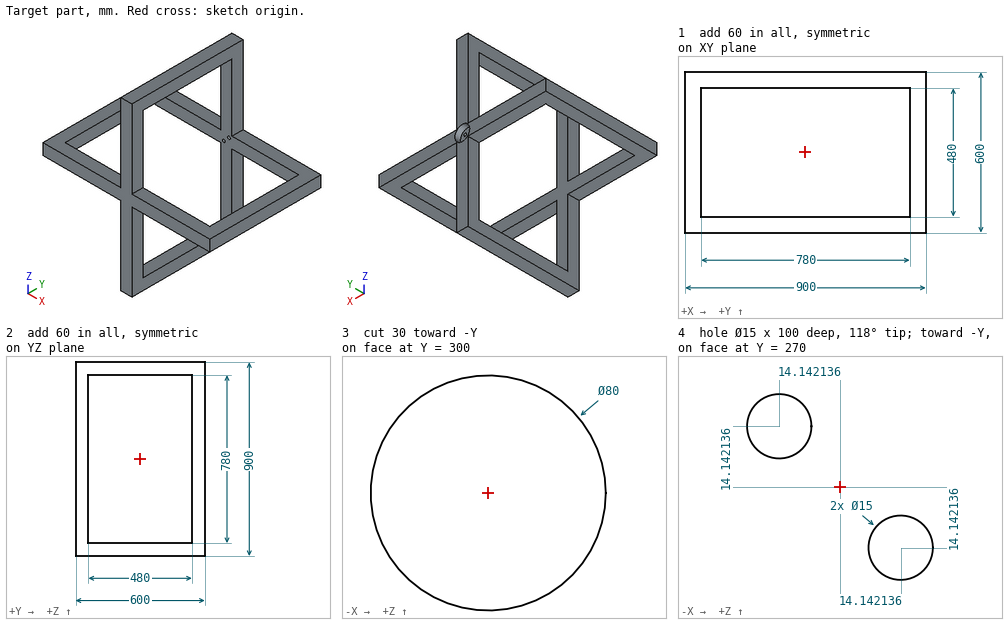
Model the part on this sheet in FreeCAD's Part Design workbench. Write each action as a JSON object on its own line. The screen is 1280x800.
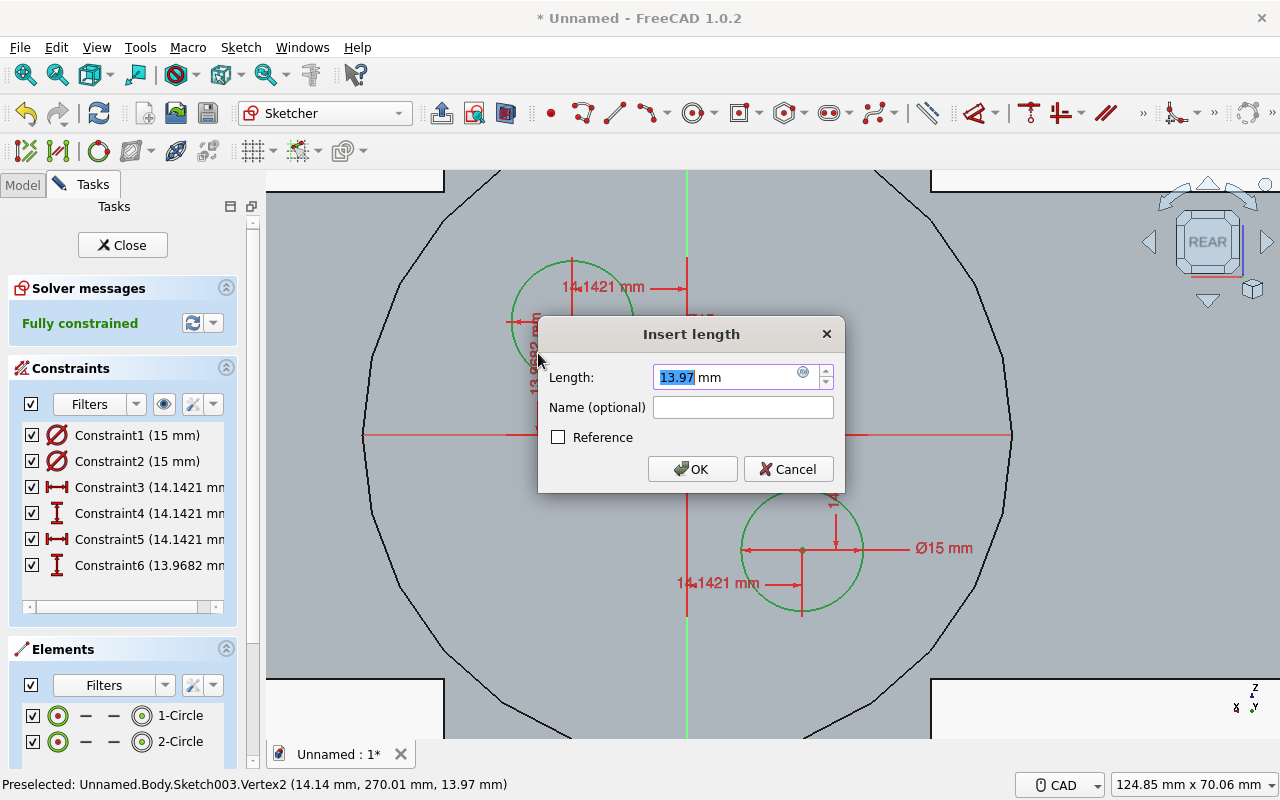
{"action": "type", "text": "14.142136"}
{"action": "key", "text": "Return"}
{"action": "key", "text": "Escape"}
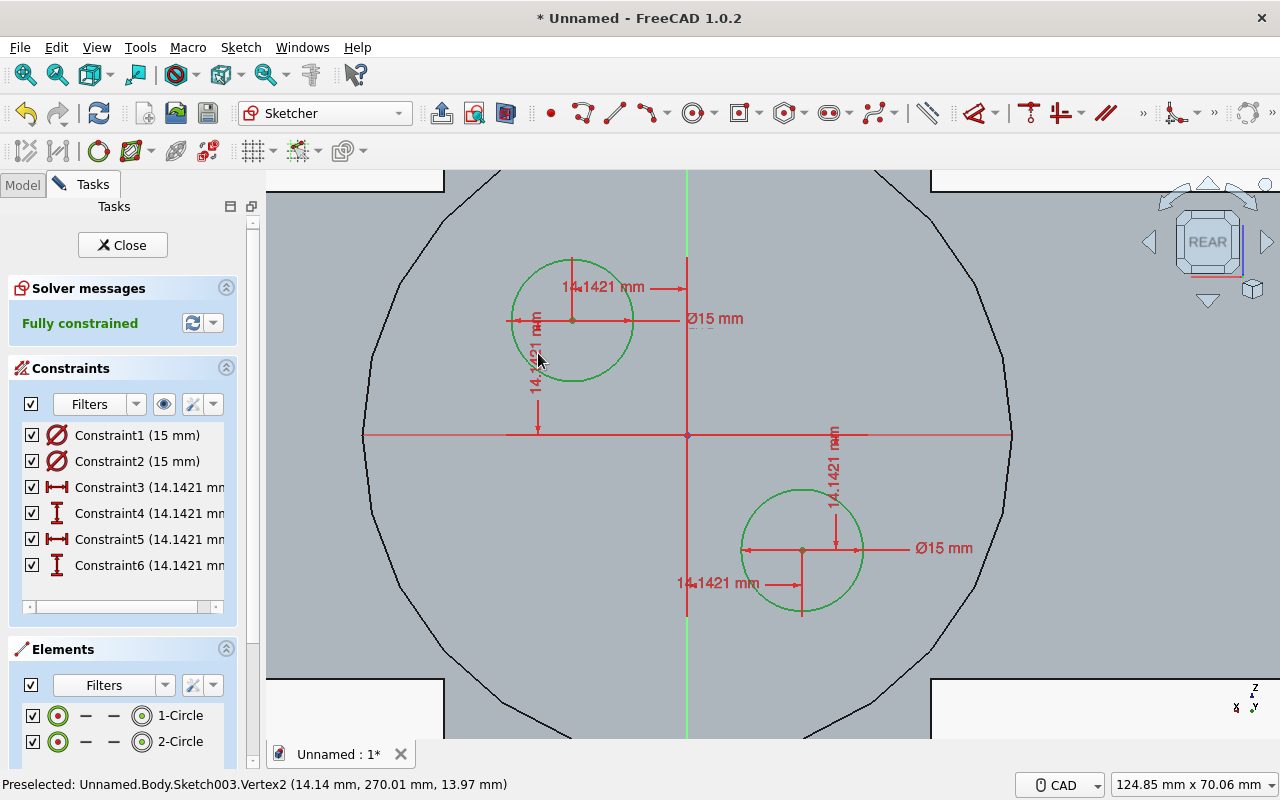
{"action": "left_click", "coordinate": [123, 245]}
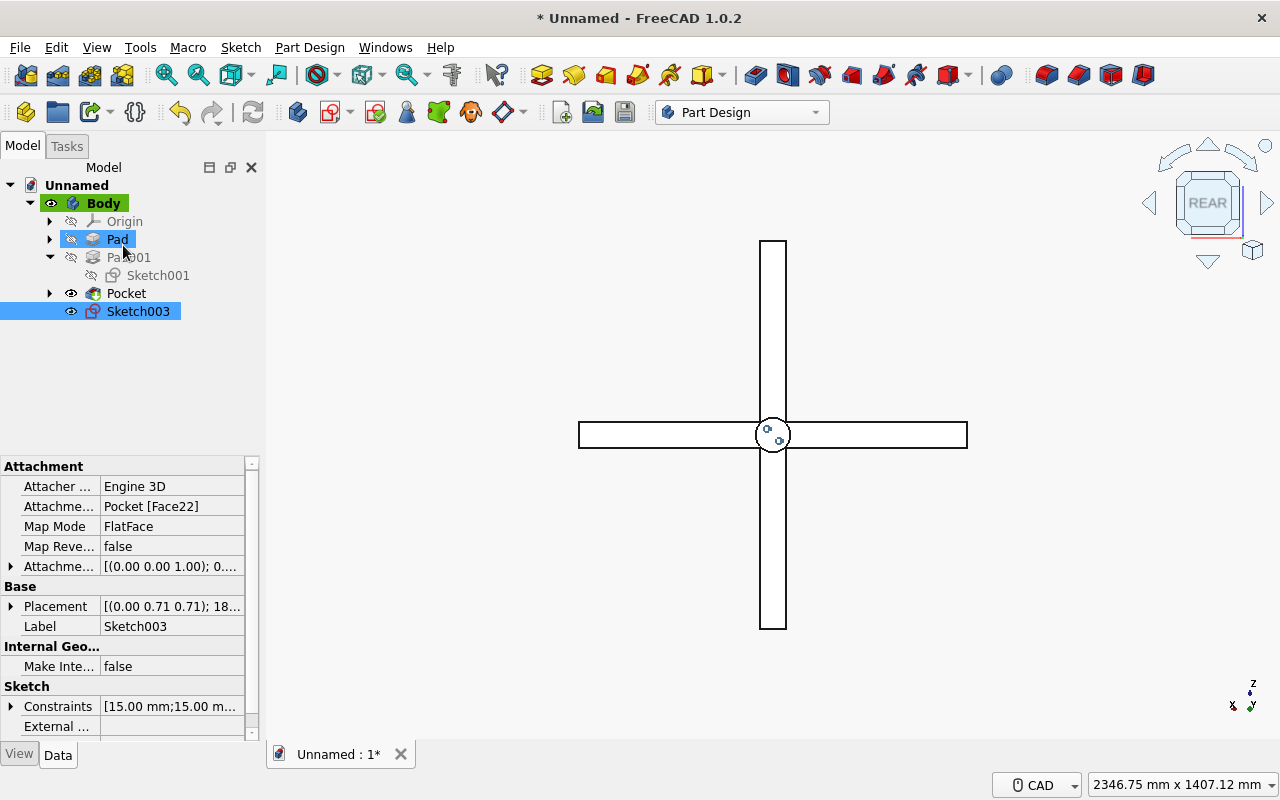
{"action": "left_click", "coordinate": [788, 76]}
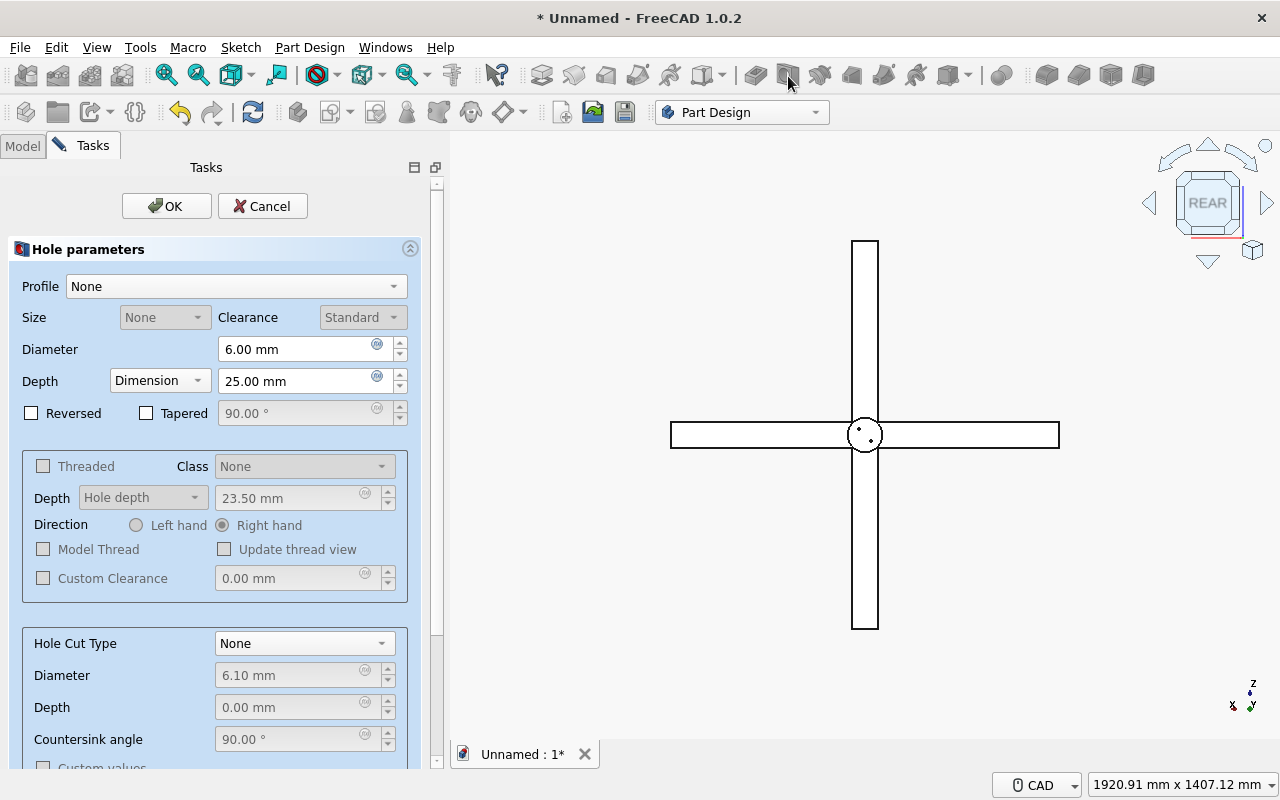
{"action": "triple_click", "coordinate": [305, 349]}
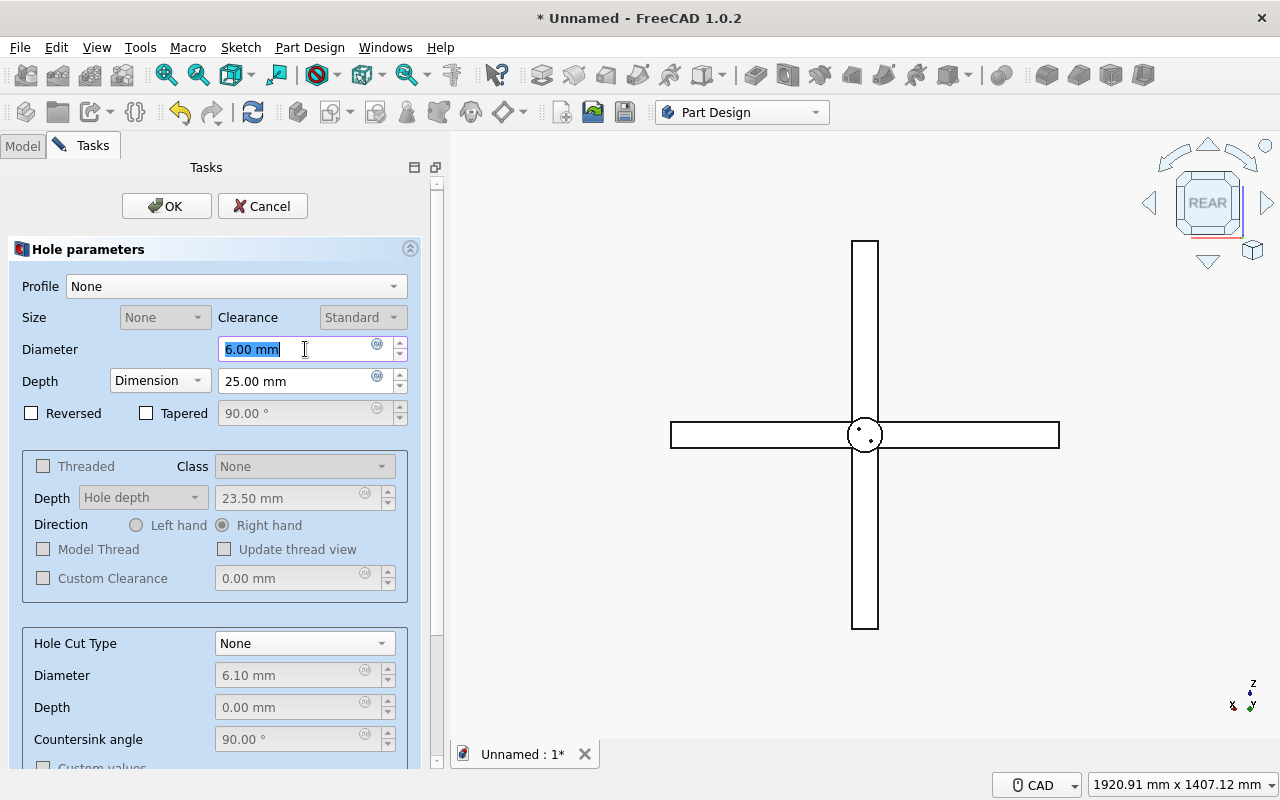
{"action": "type", "text": "15"}
{"action": "key", "text": "Tab"}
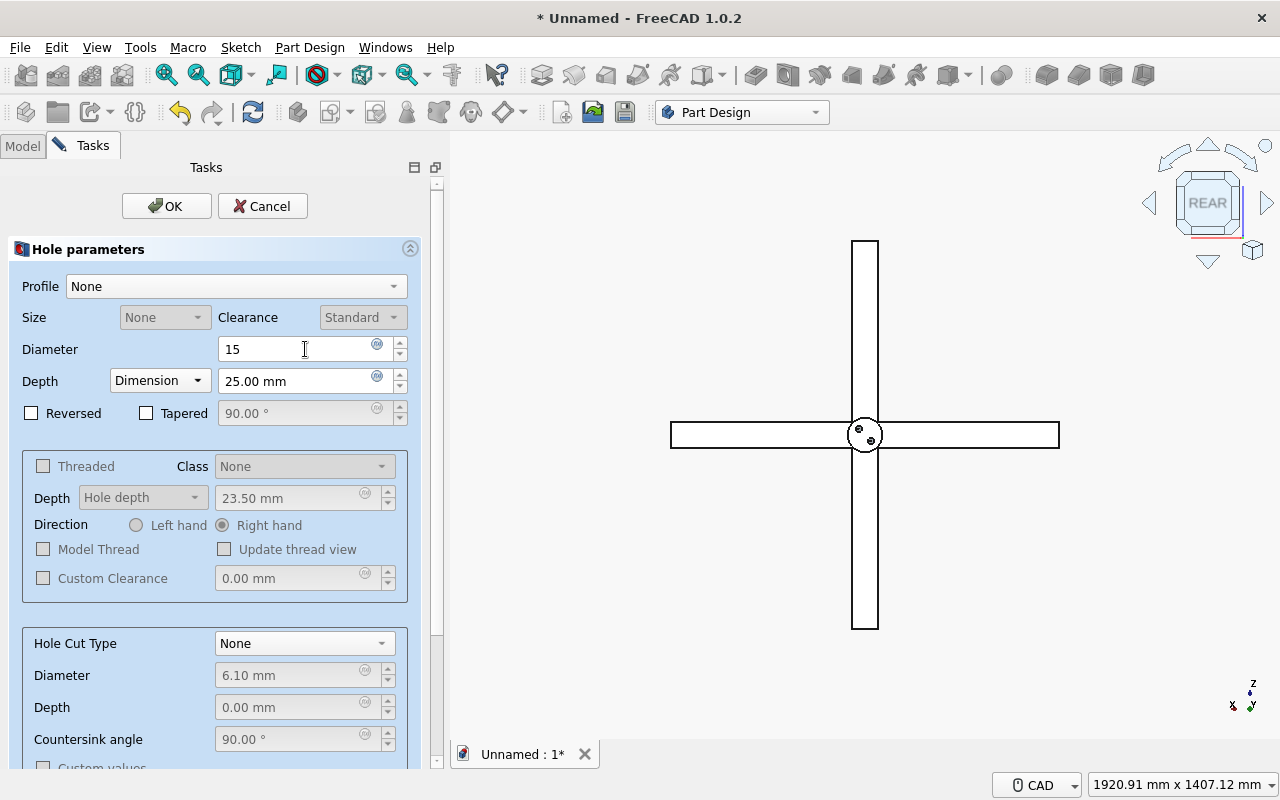
{"action": "triple_click", "coordinate": [305, 381]}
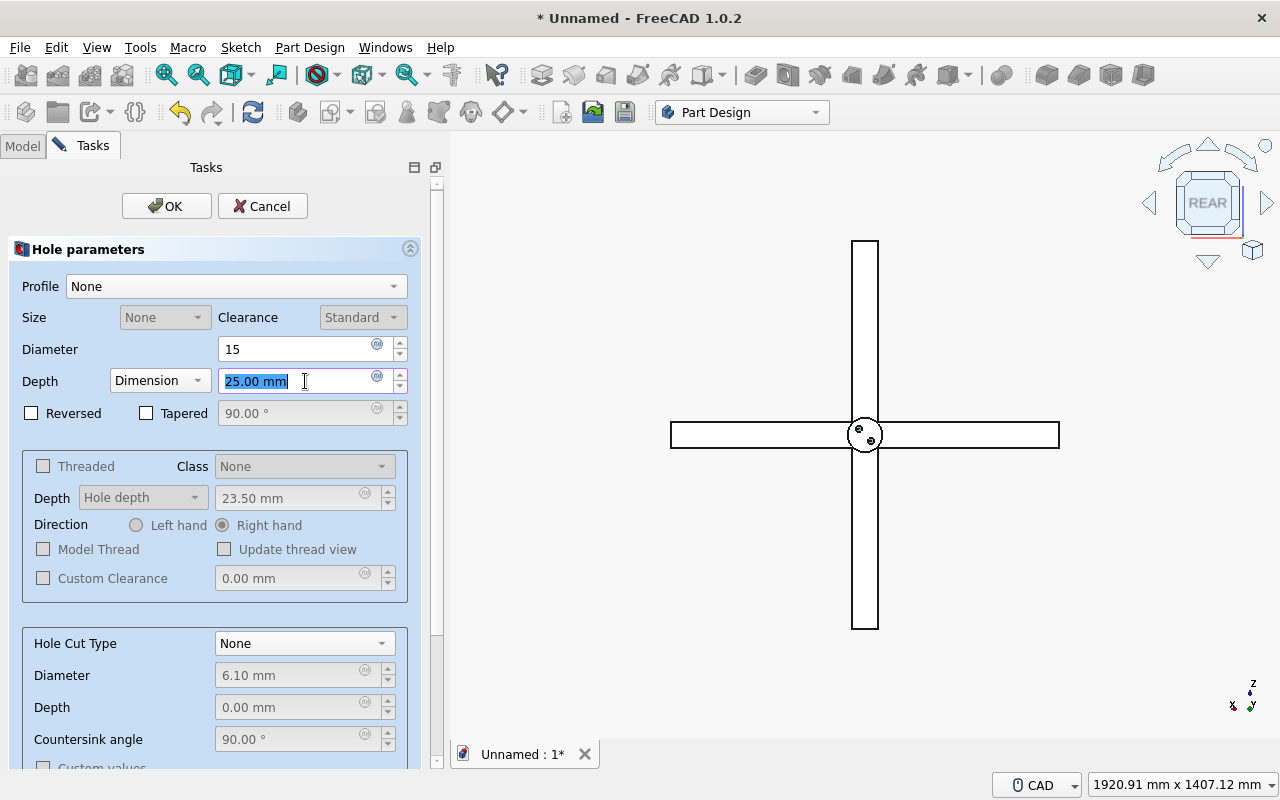
{"action": "type", "text": "100"}
{"action": "key", "text": "Tab"}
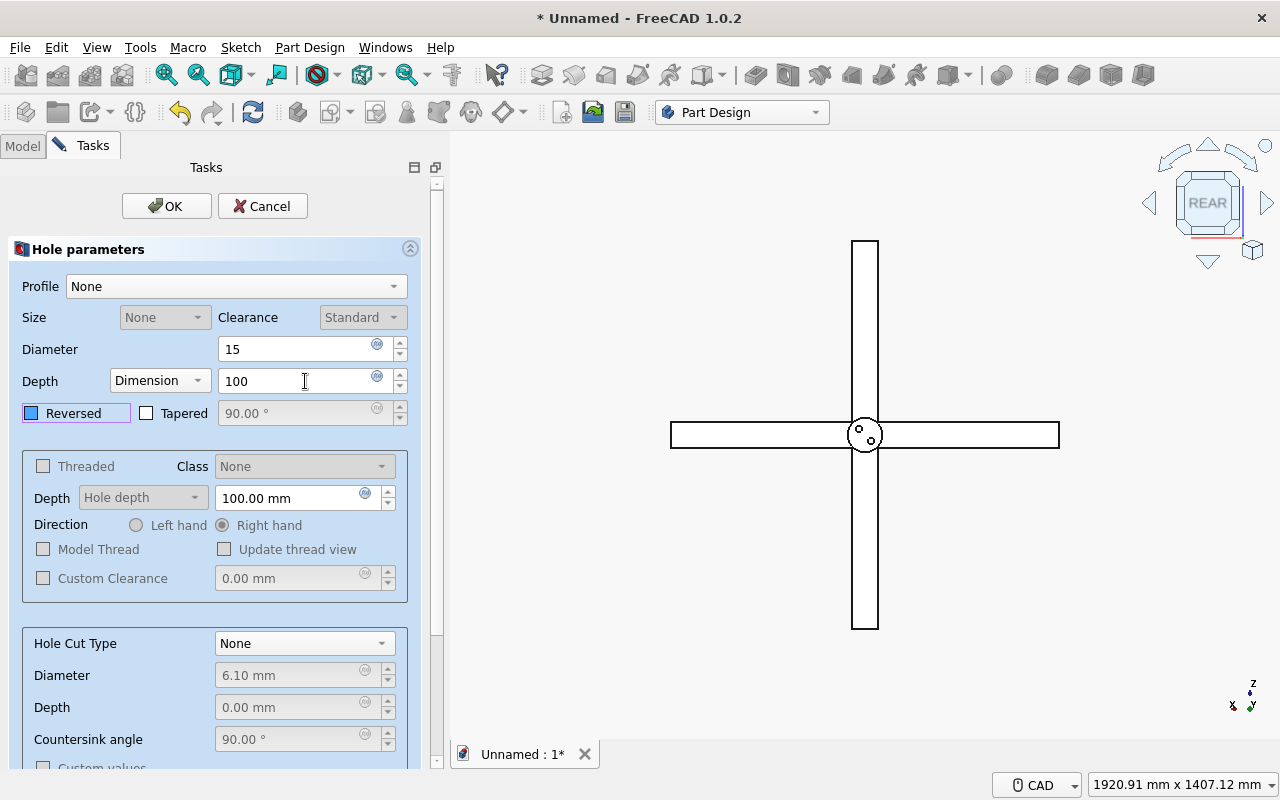
{"action": "left_click", "coordinate": [167, 206]}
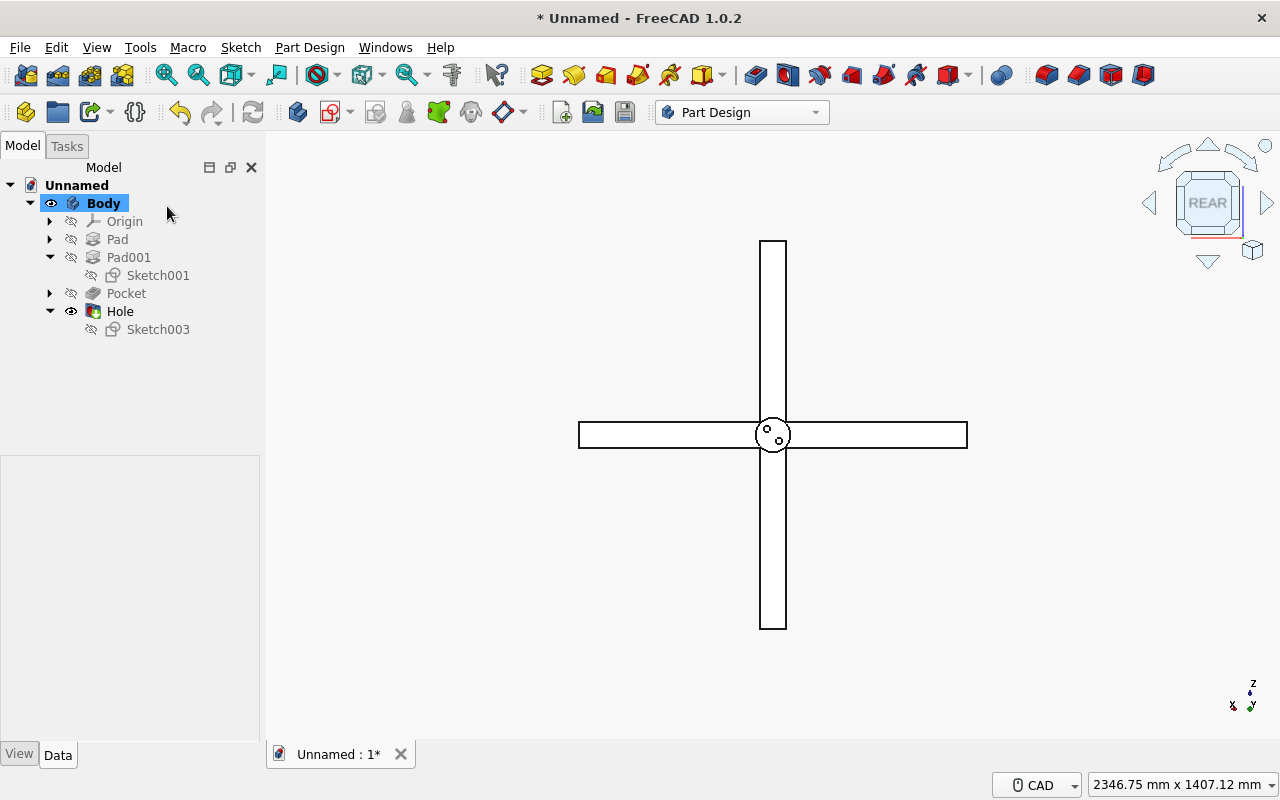
{"action": "key", "text": "0"}